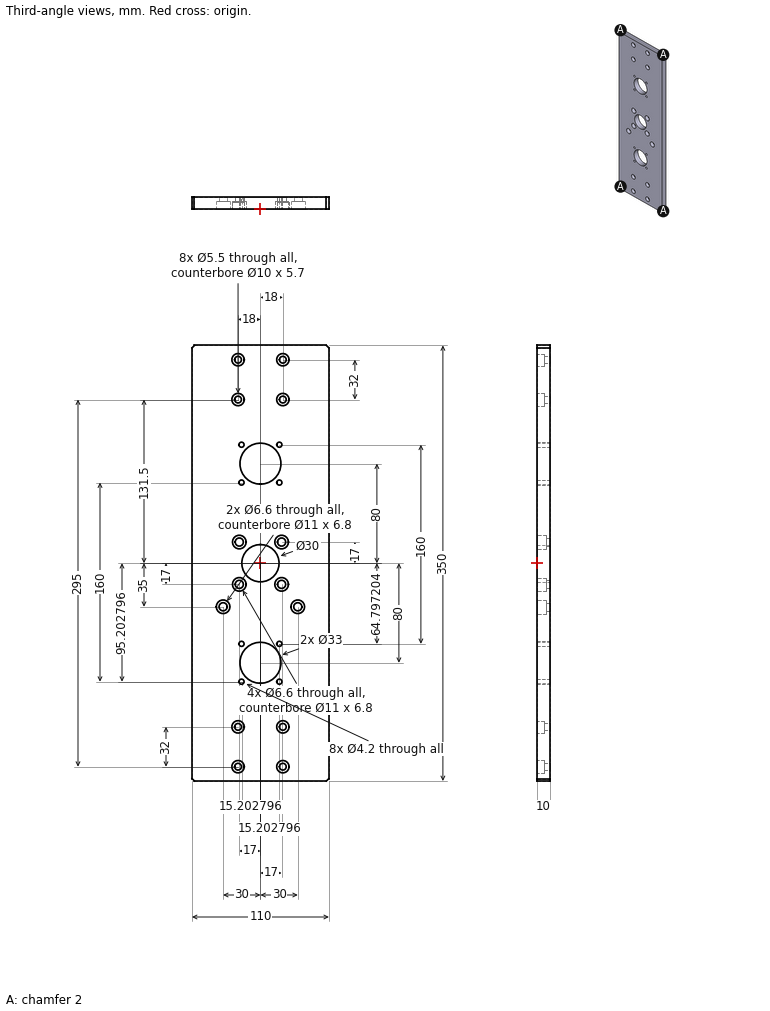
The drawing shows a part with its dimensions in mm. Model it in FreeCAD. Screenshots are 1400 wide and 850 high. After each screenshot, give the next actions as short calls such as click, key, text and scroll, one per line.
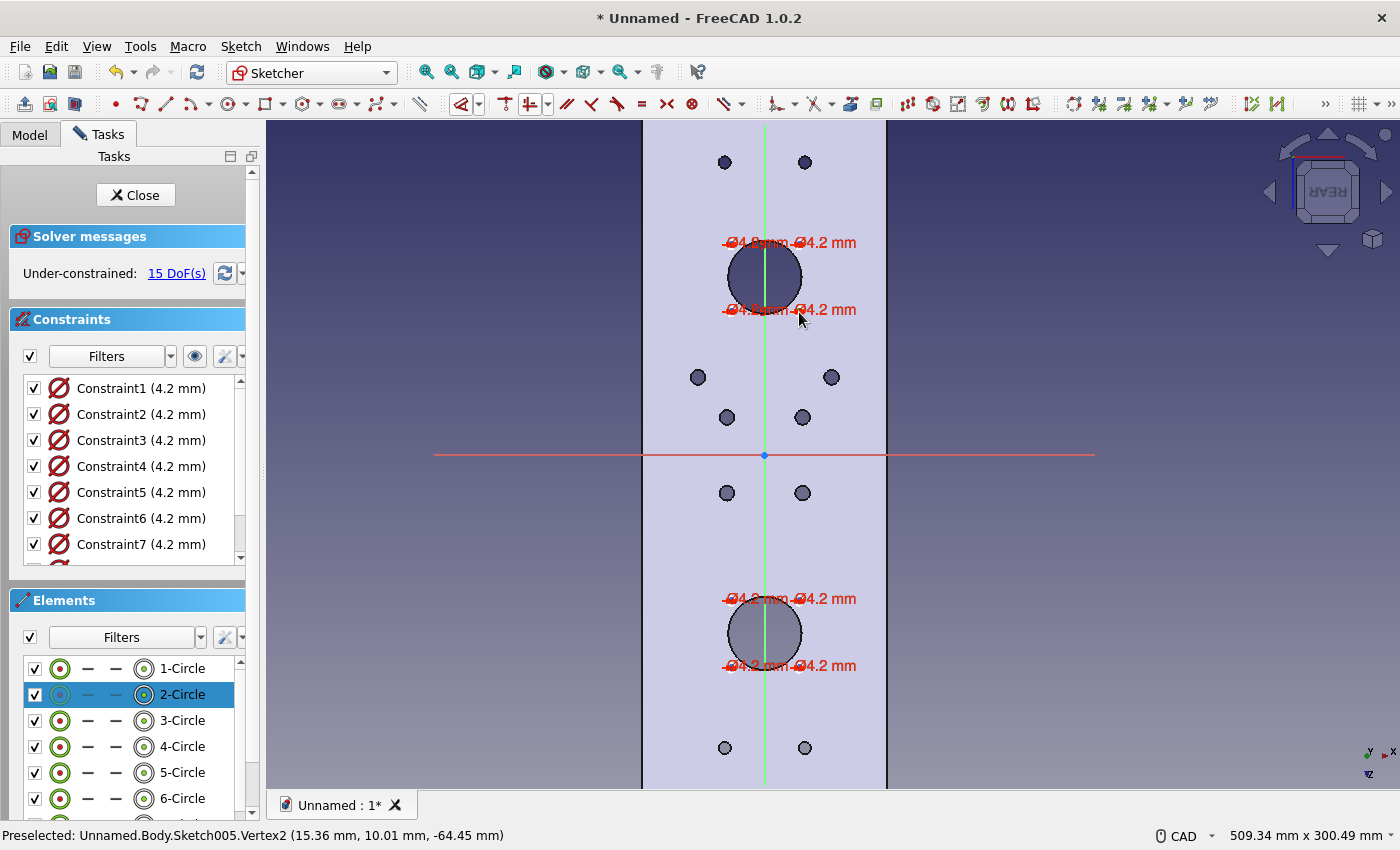
click(731, 312)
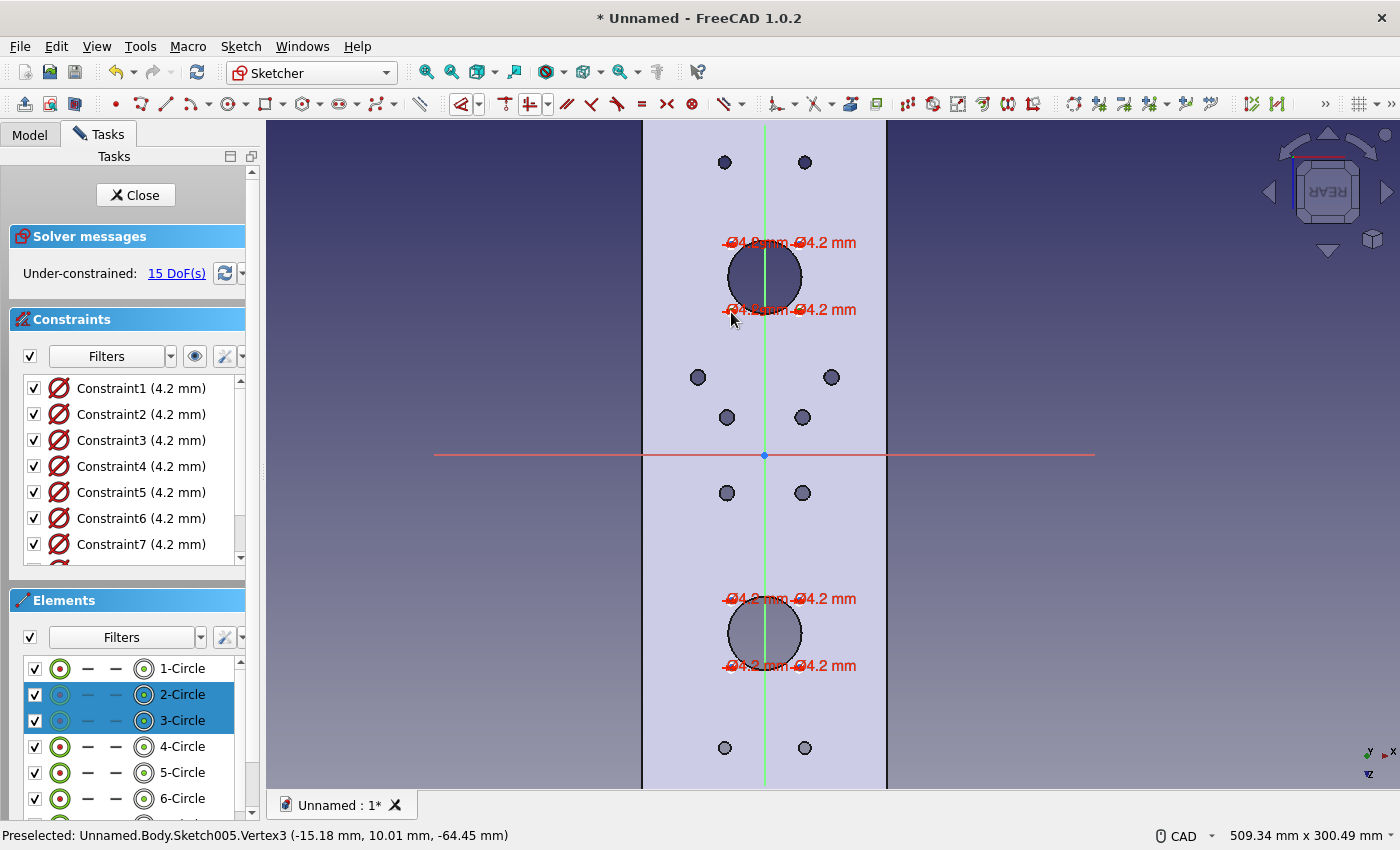
key(h)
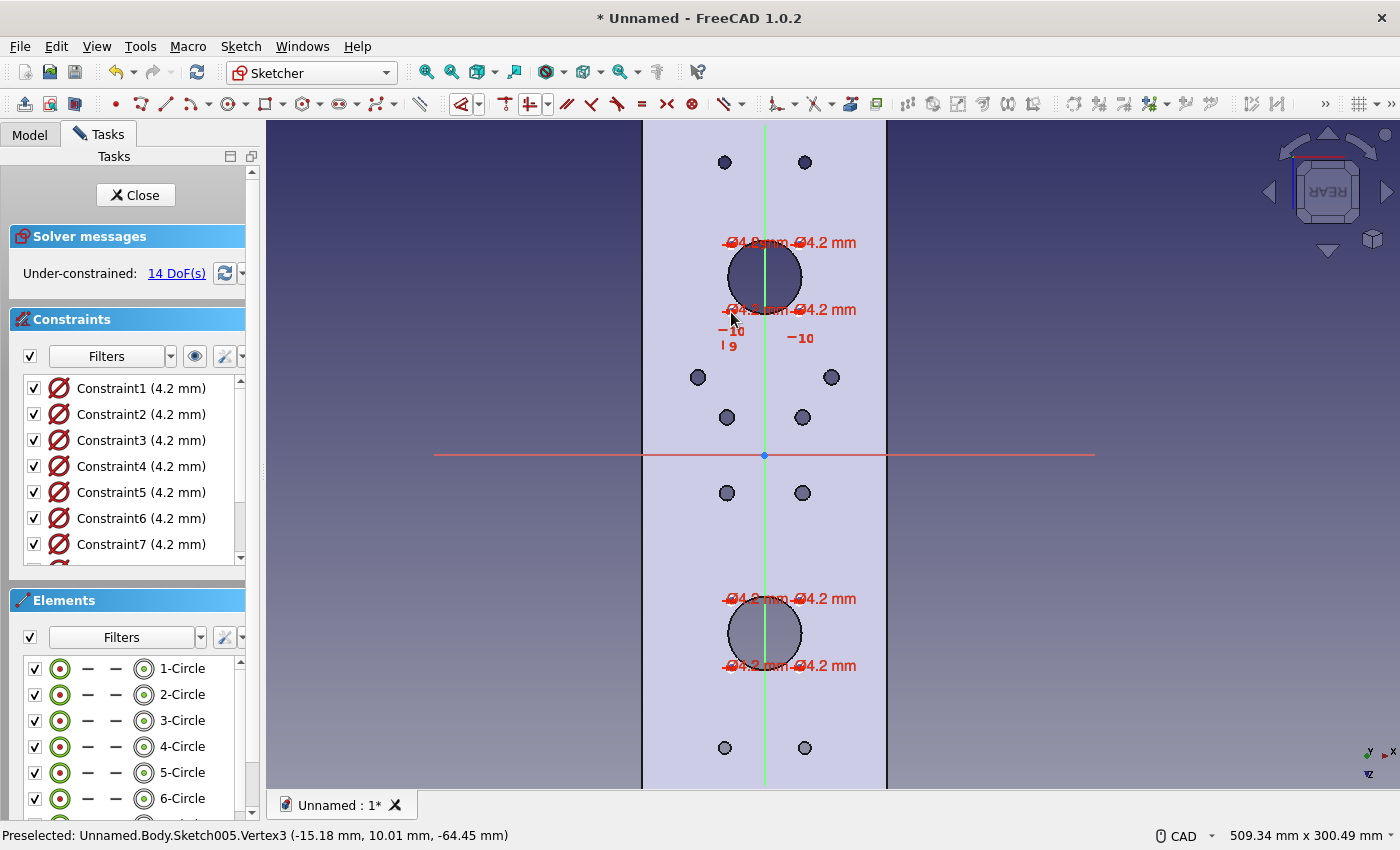
click(799, 312)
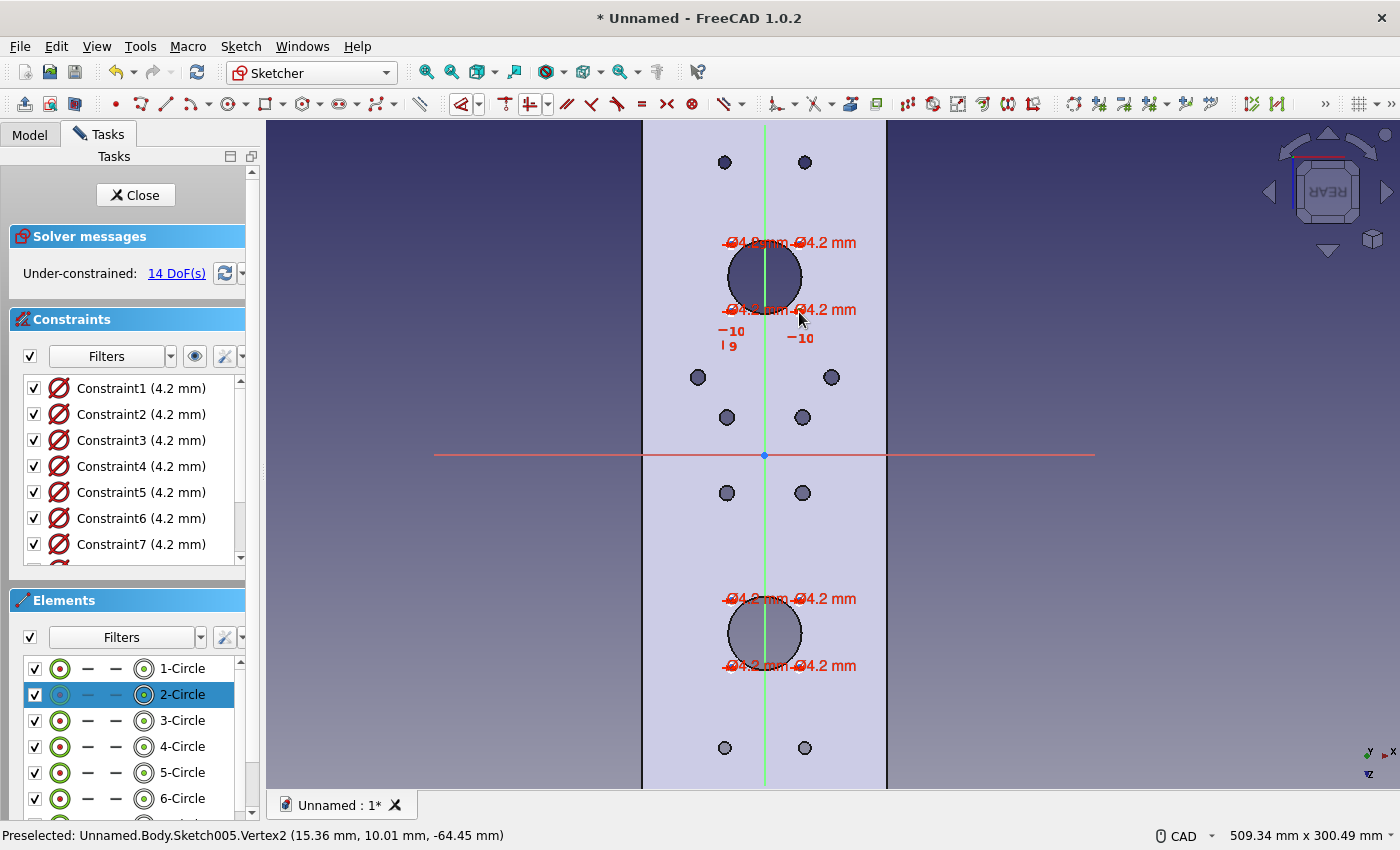
click(799, 245)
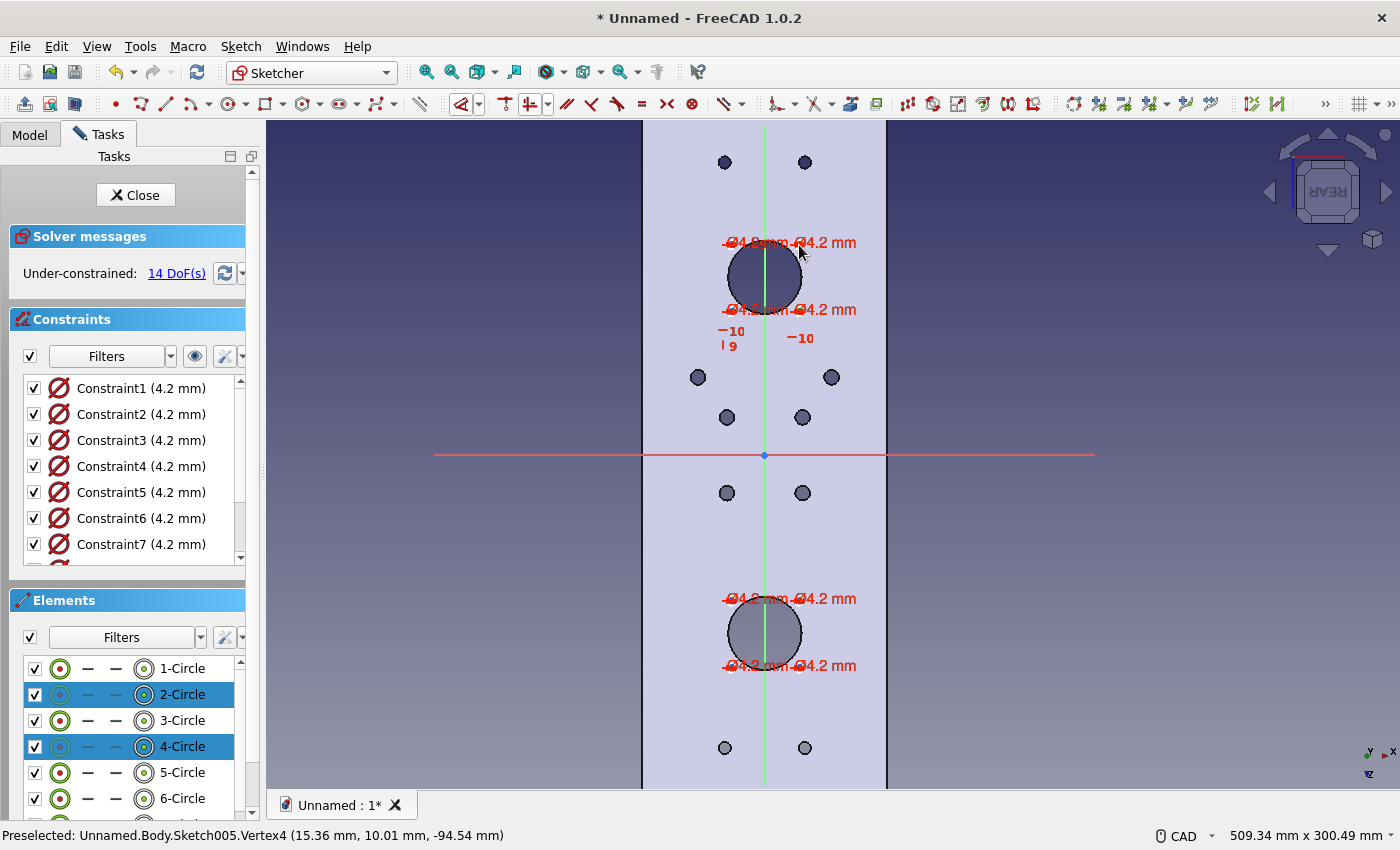
click(548, 104)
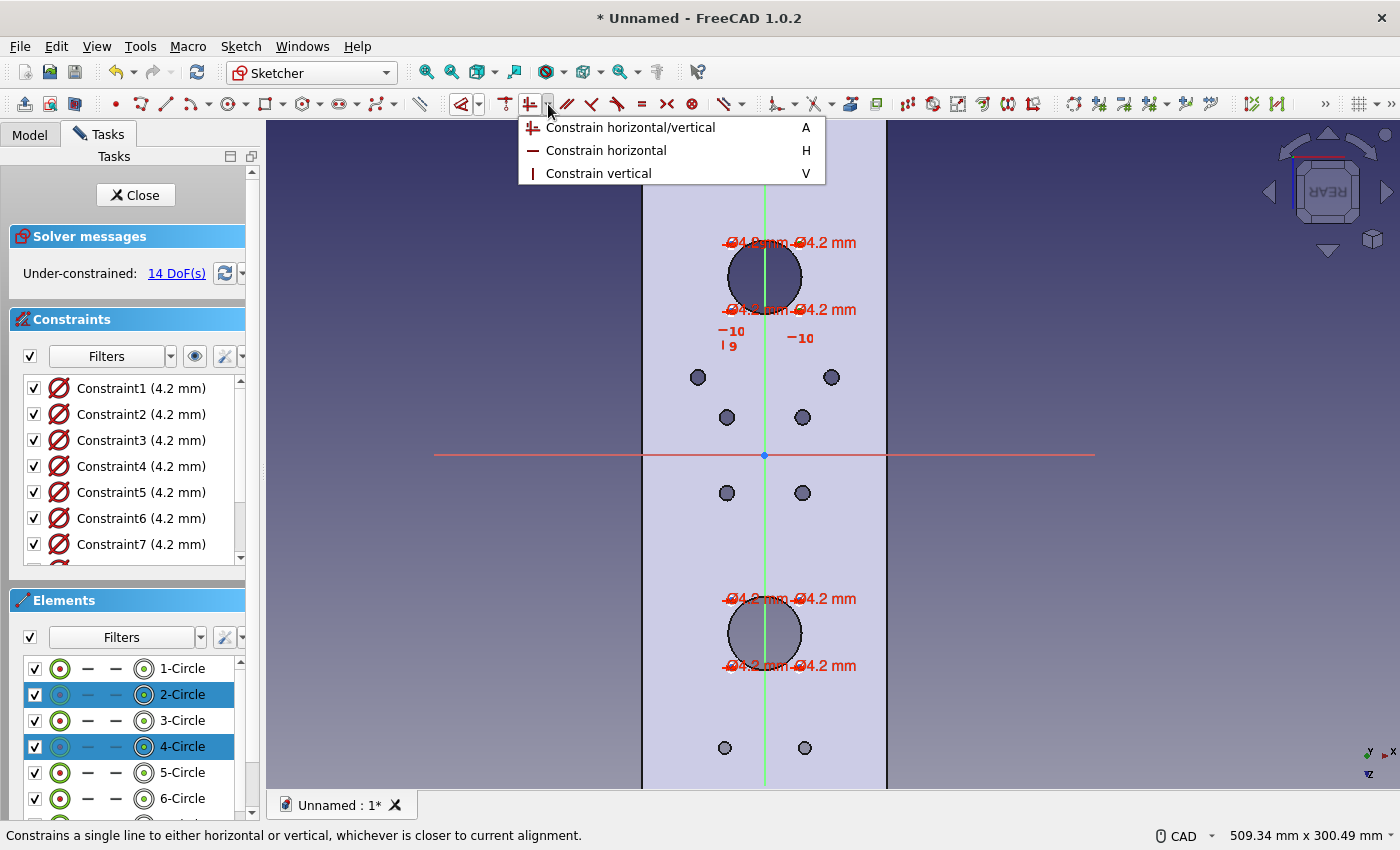
click(672, 174)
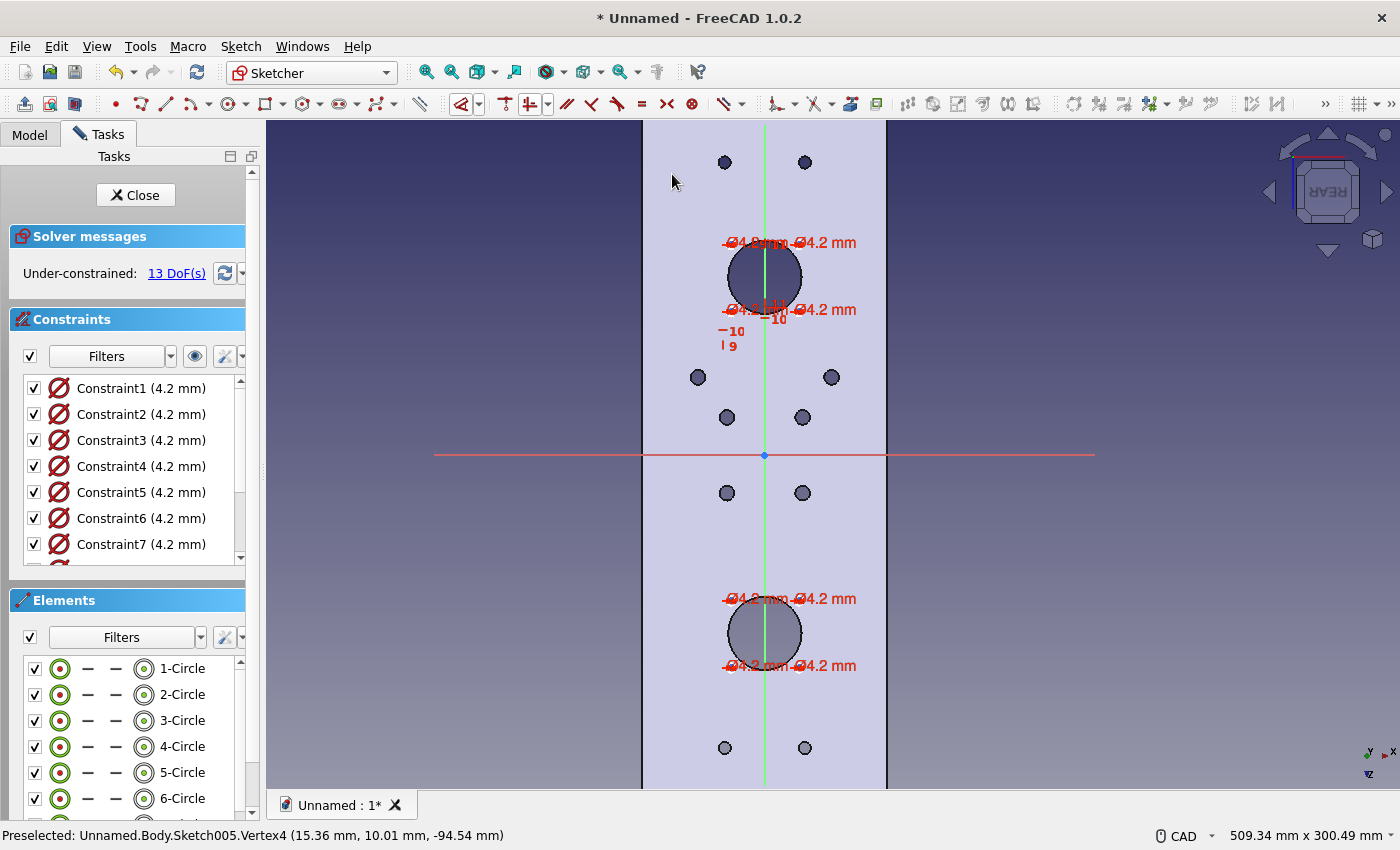
click(731, 245)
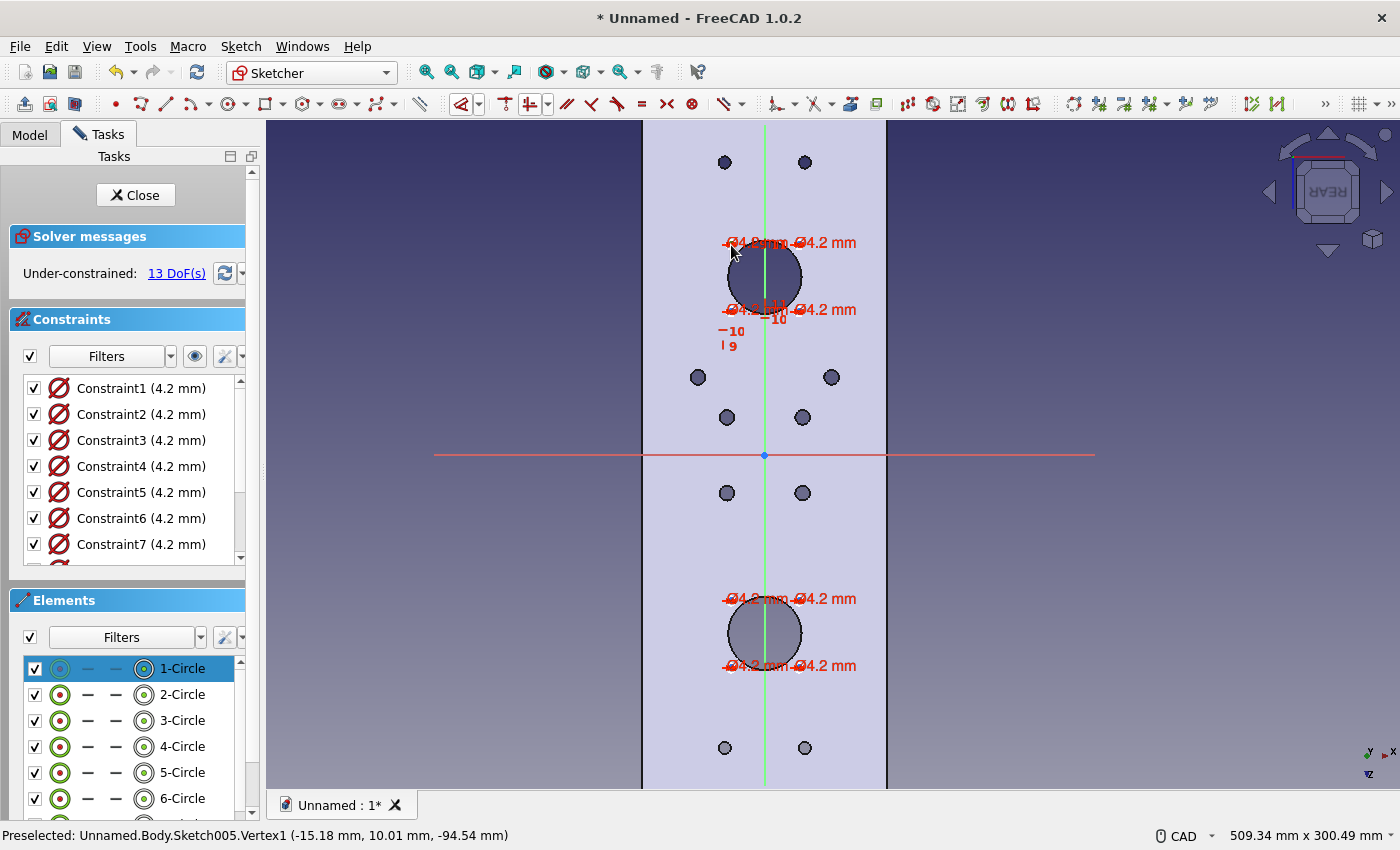
click(799, 245)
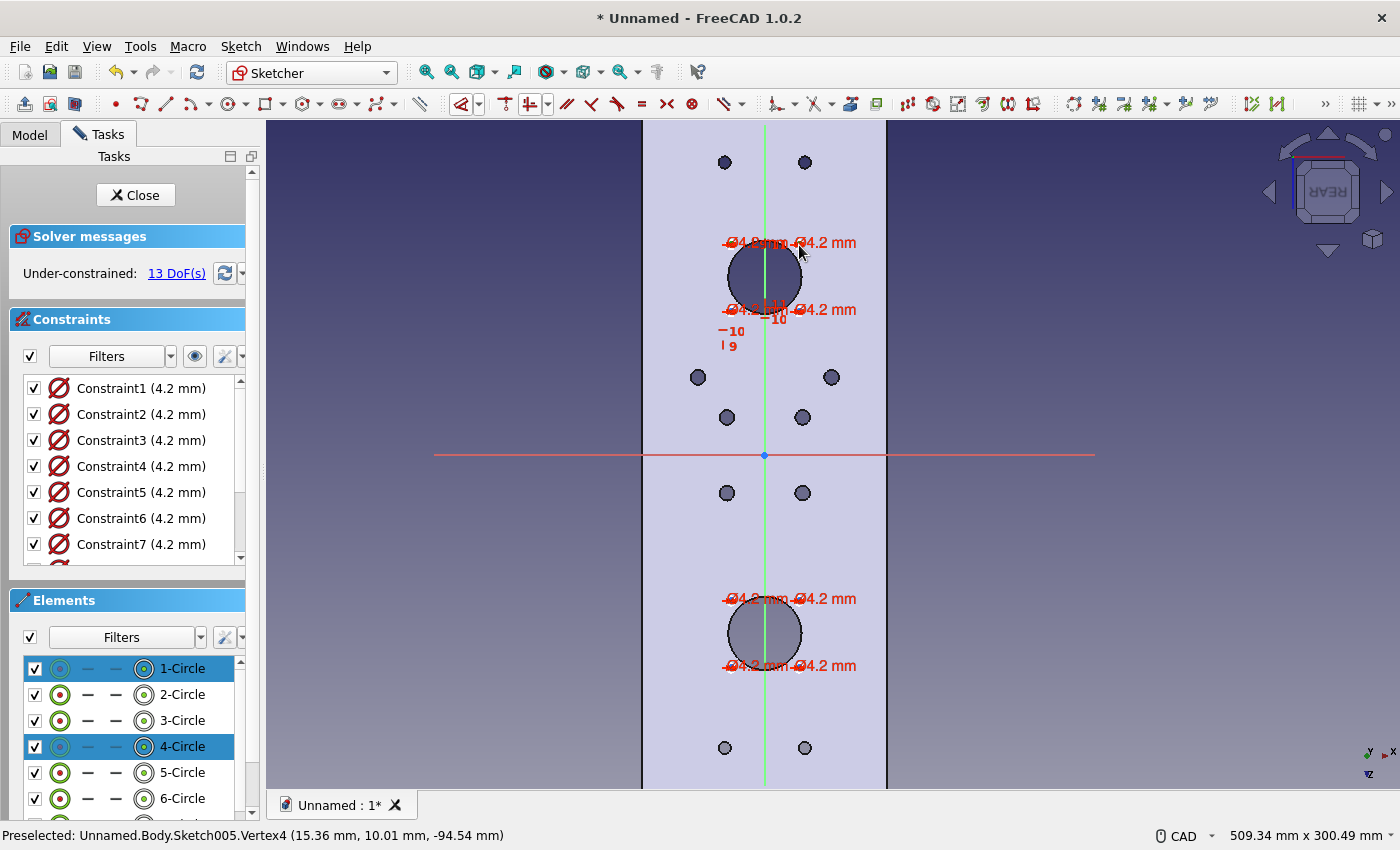
key(h)